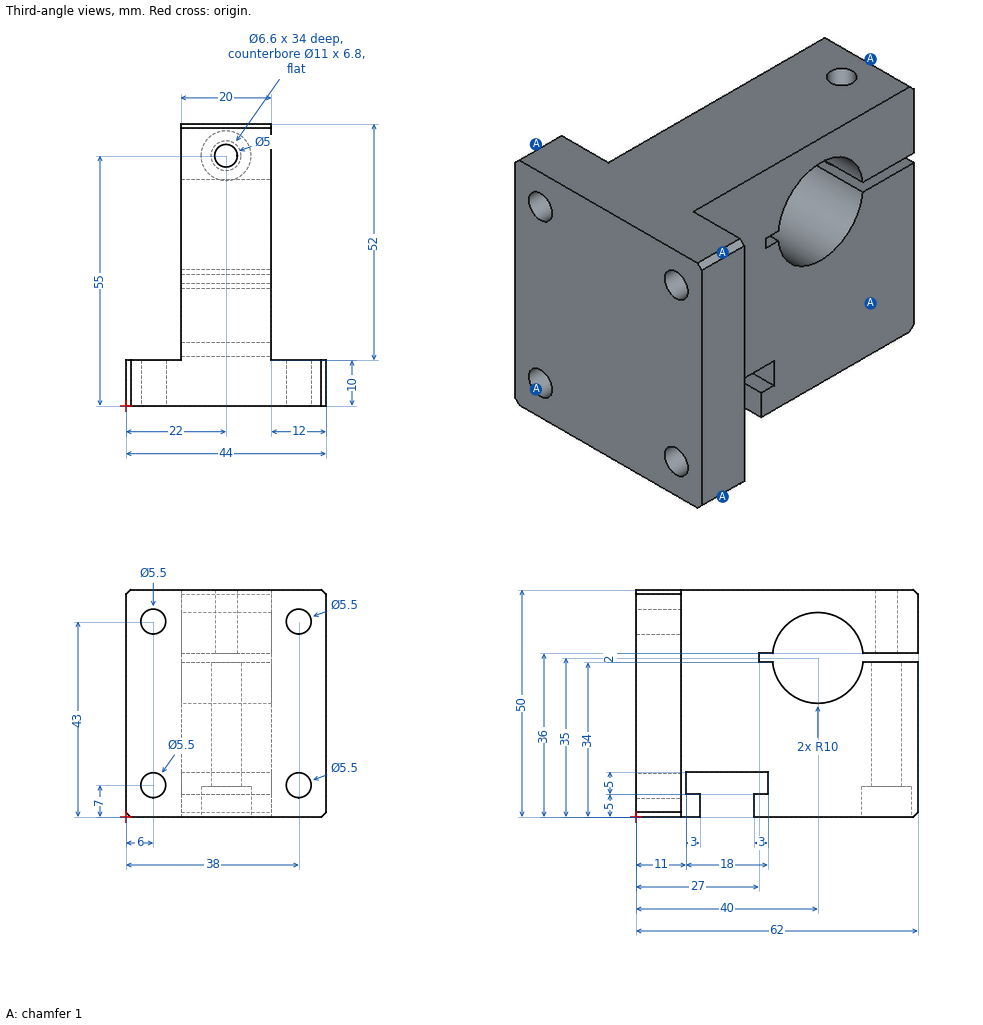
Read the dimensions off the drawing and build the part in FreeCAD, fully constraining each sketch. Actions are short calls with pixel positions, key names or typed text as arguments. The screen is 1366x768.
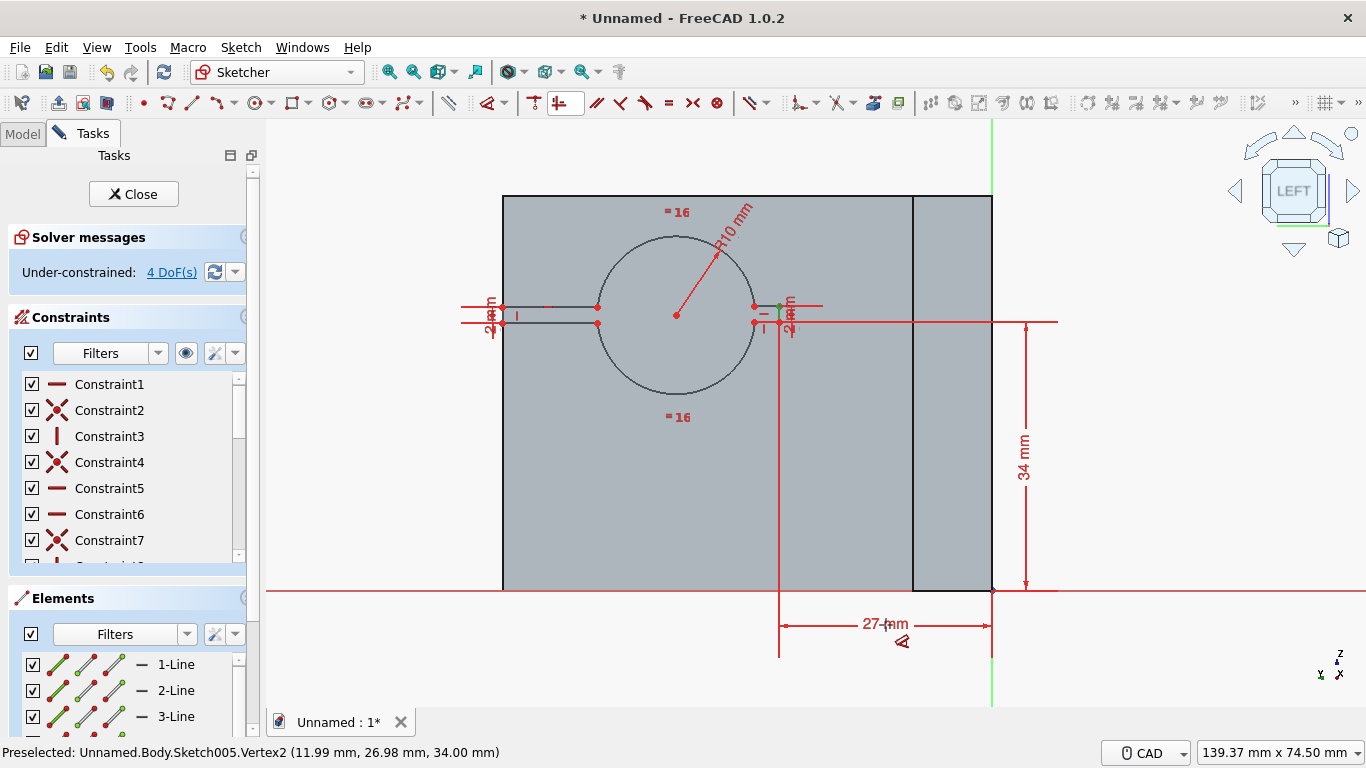
click(598, 307)
click(1026, 384)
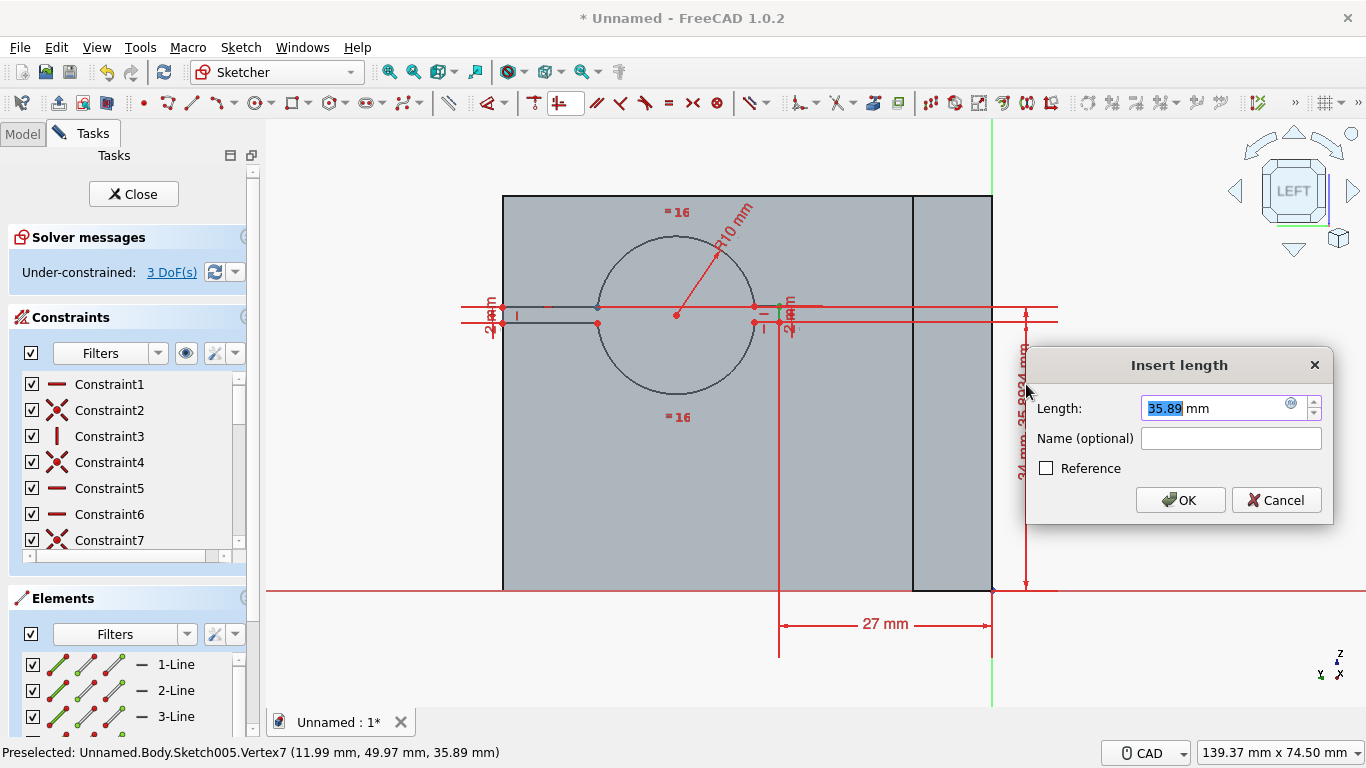
text(36)
key(Return)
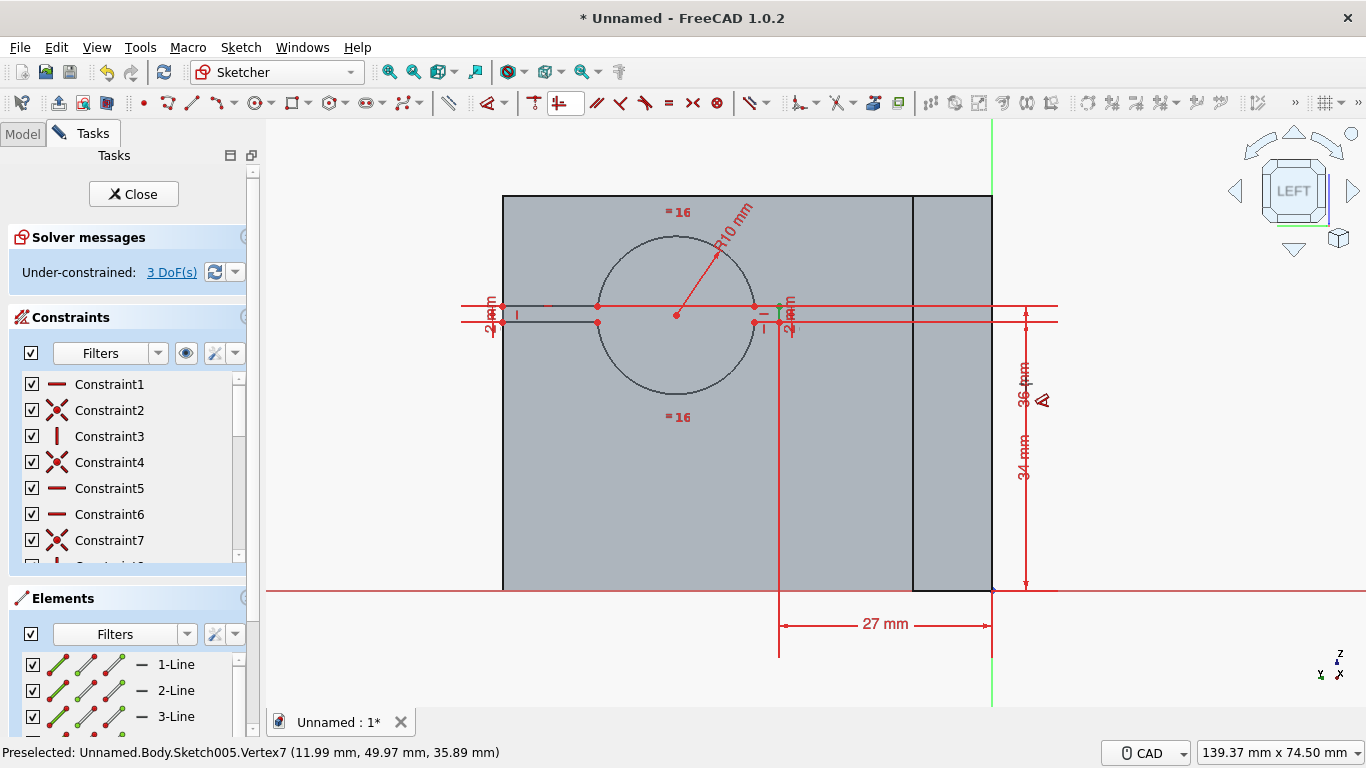
click(503, 306)
click(747, 625)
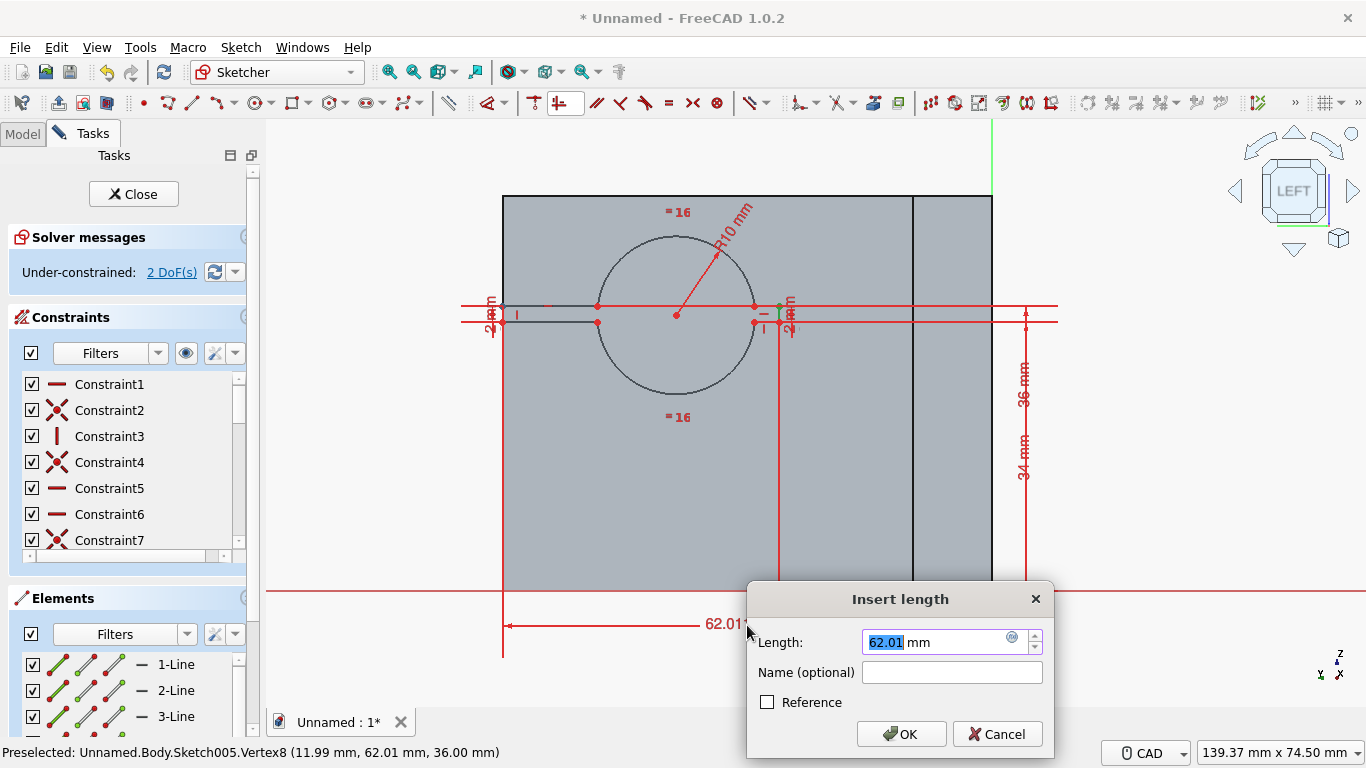
text(62)
key(Return)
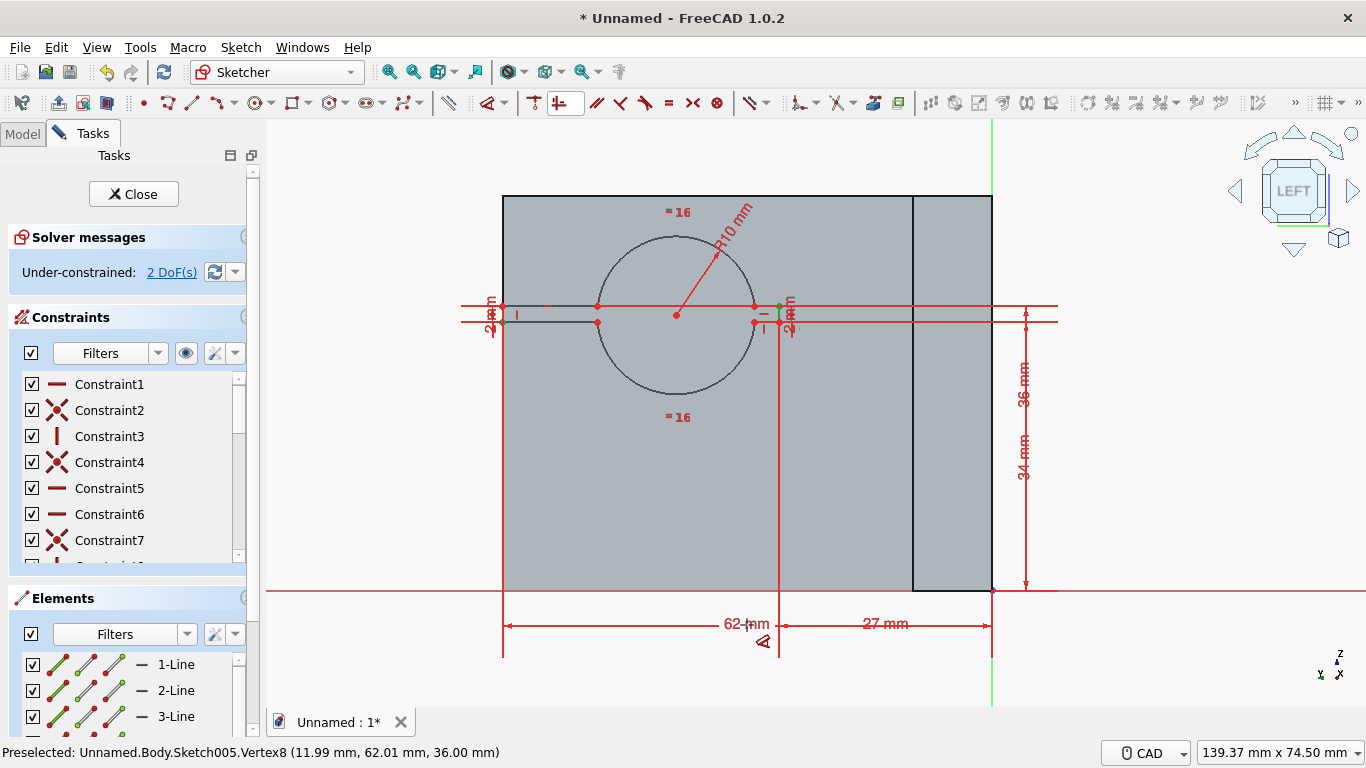
click(676, 315)
click(834, 281)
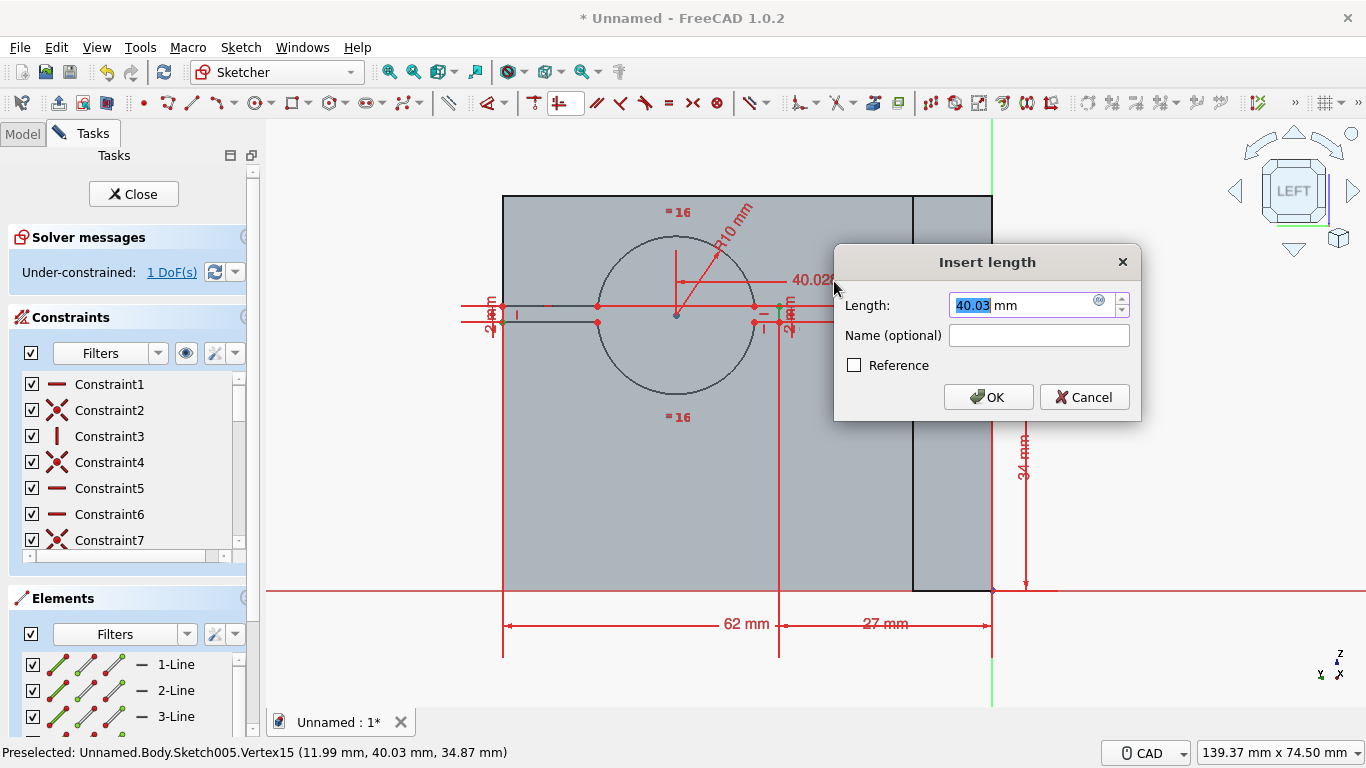
text(40)
key(Return)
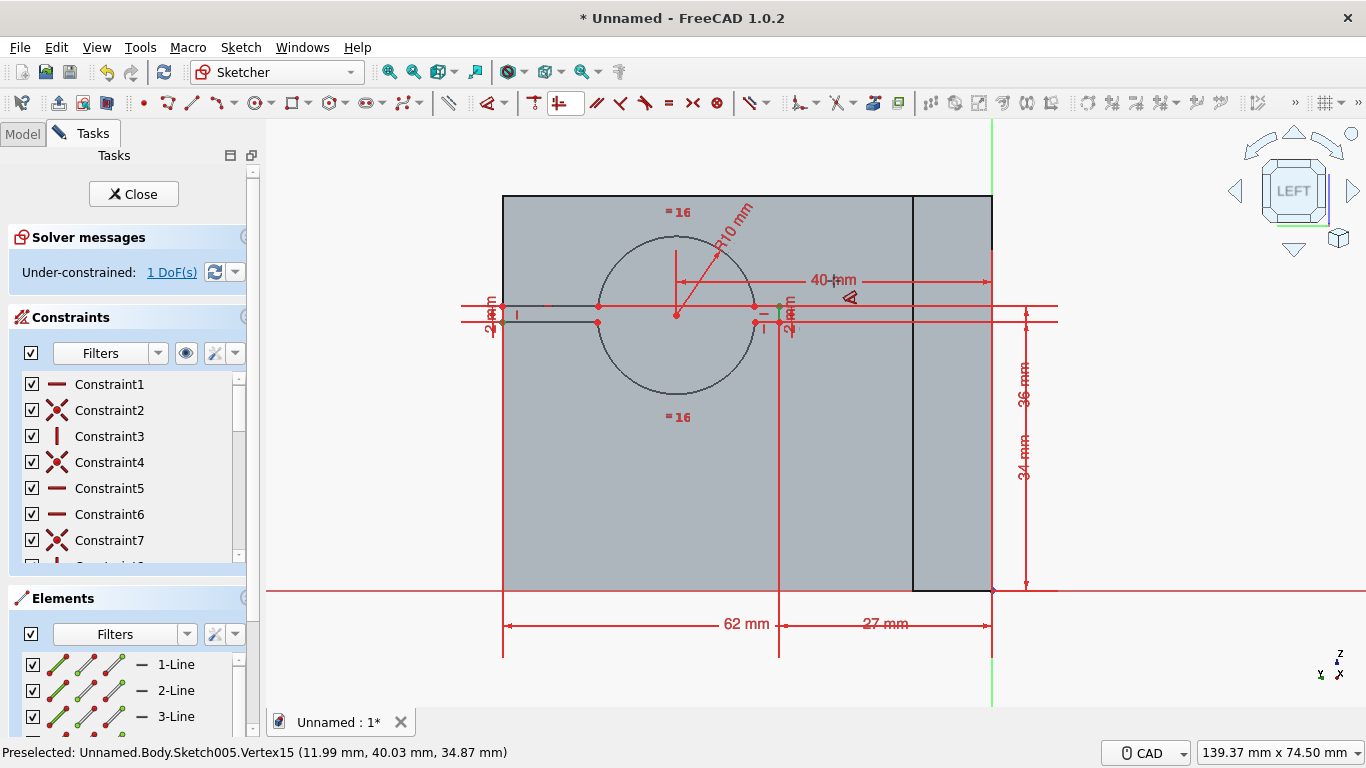
click(676, 315)
click(1026, 516)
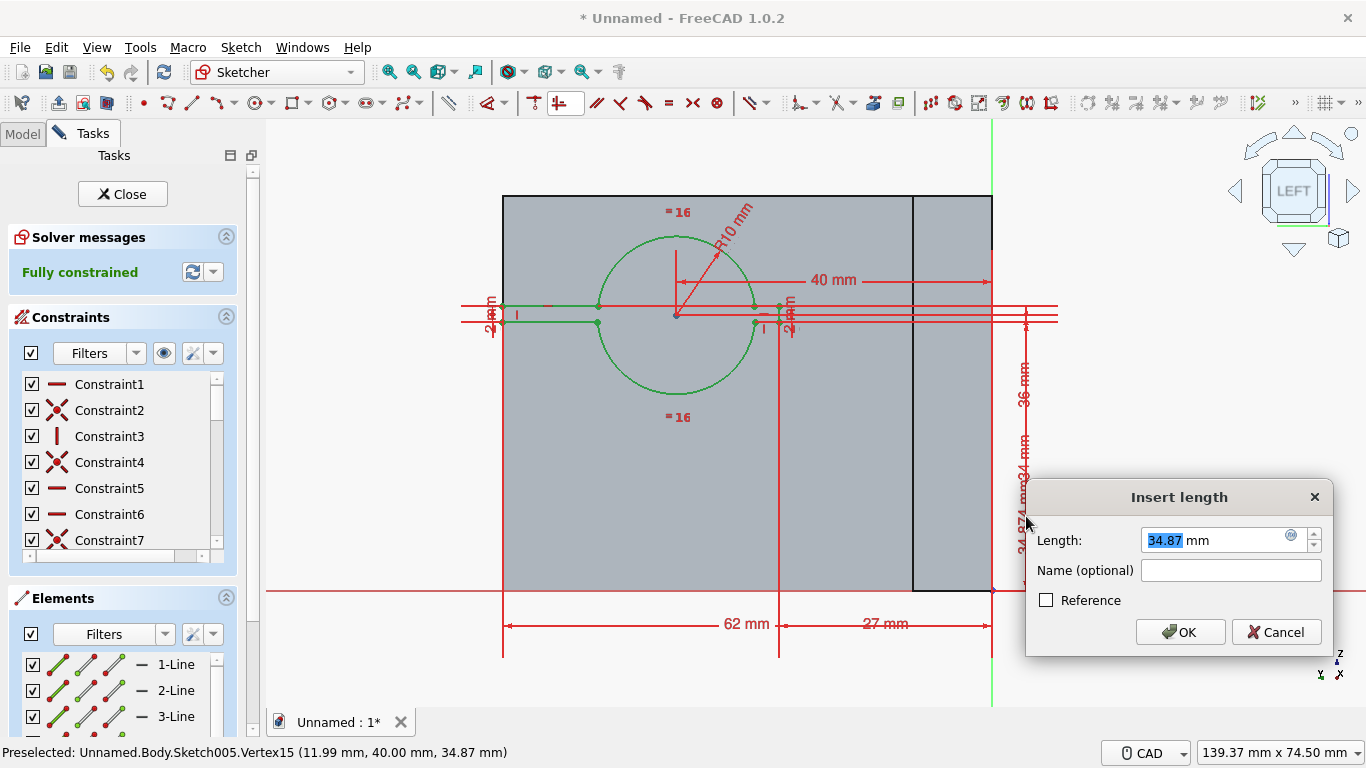
text(35)
key(Return)
key(Escape)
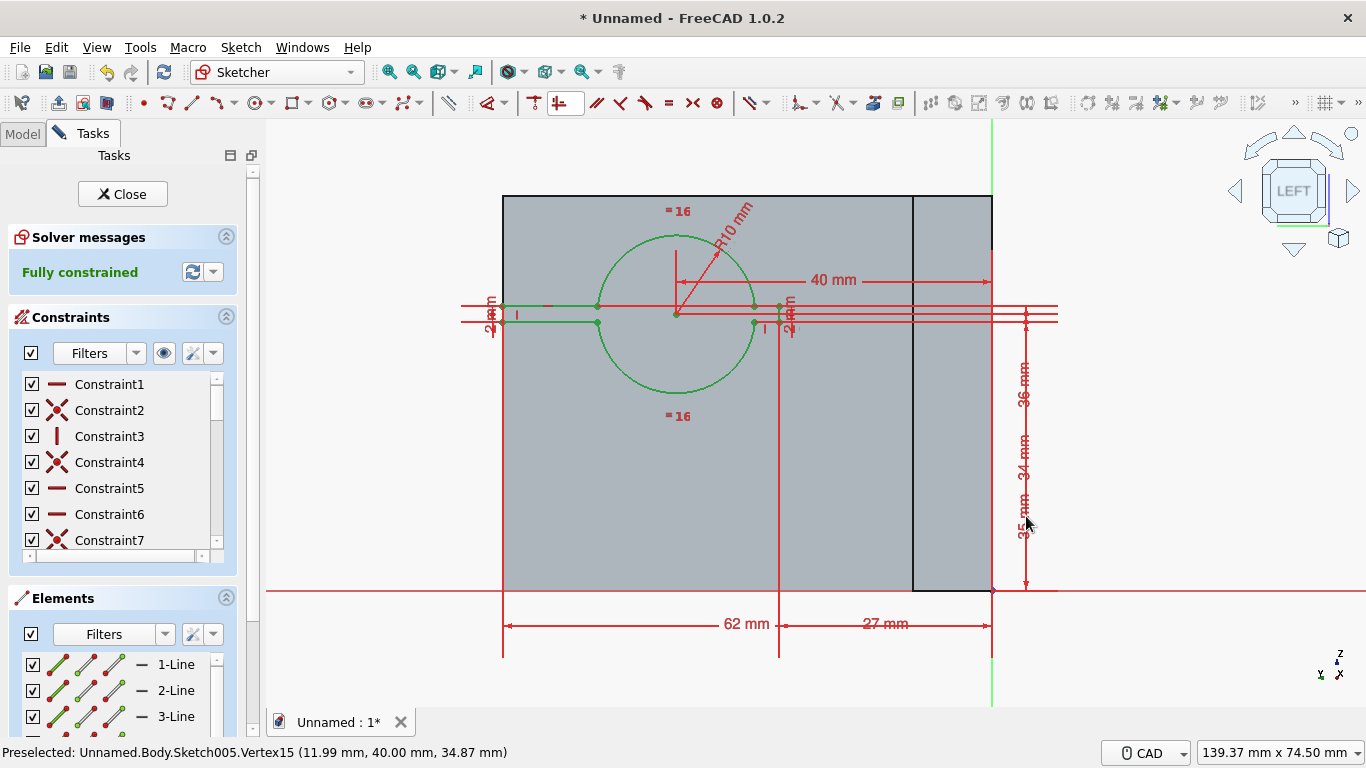
click(123, 194)